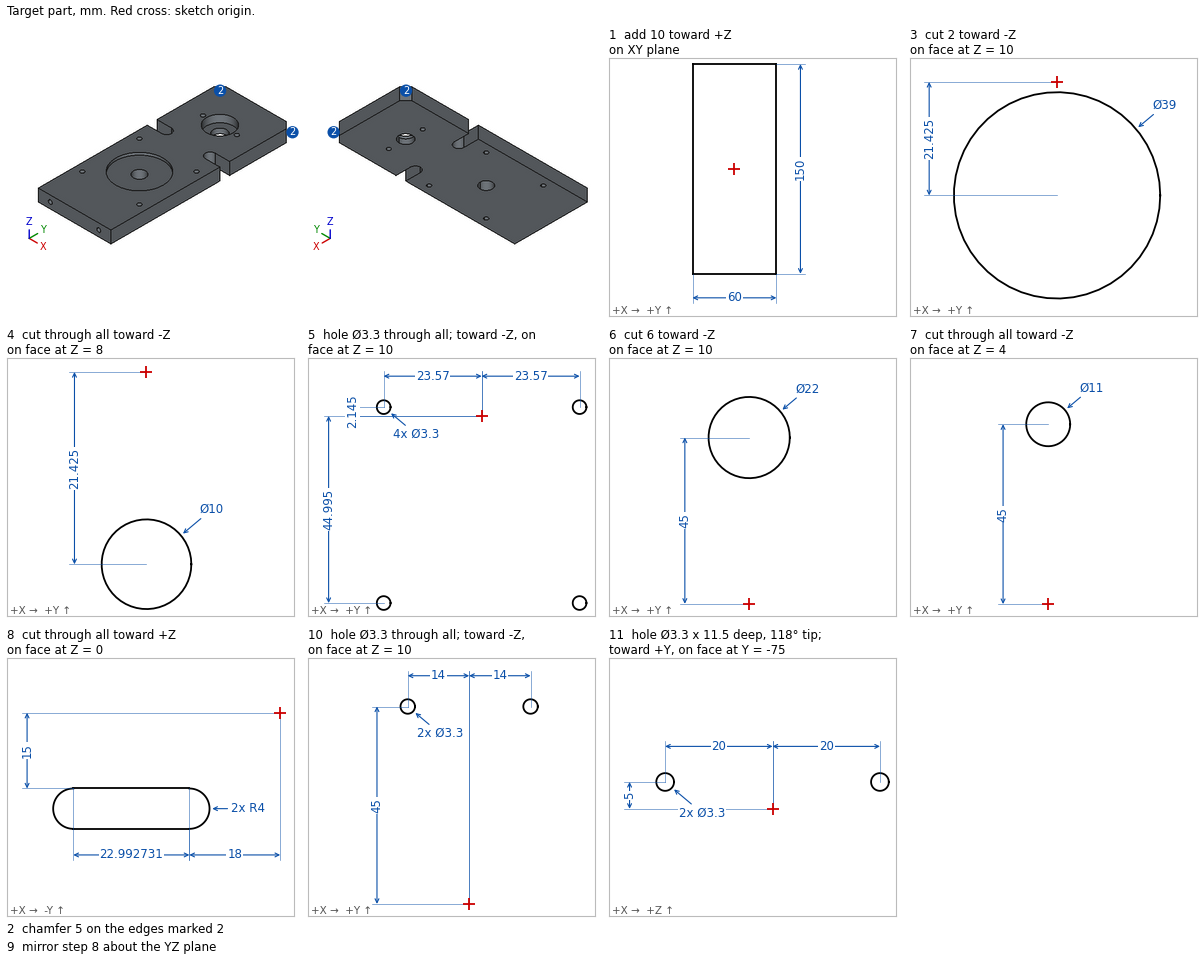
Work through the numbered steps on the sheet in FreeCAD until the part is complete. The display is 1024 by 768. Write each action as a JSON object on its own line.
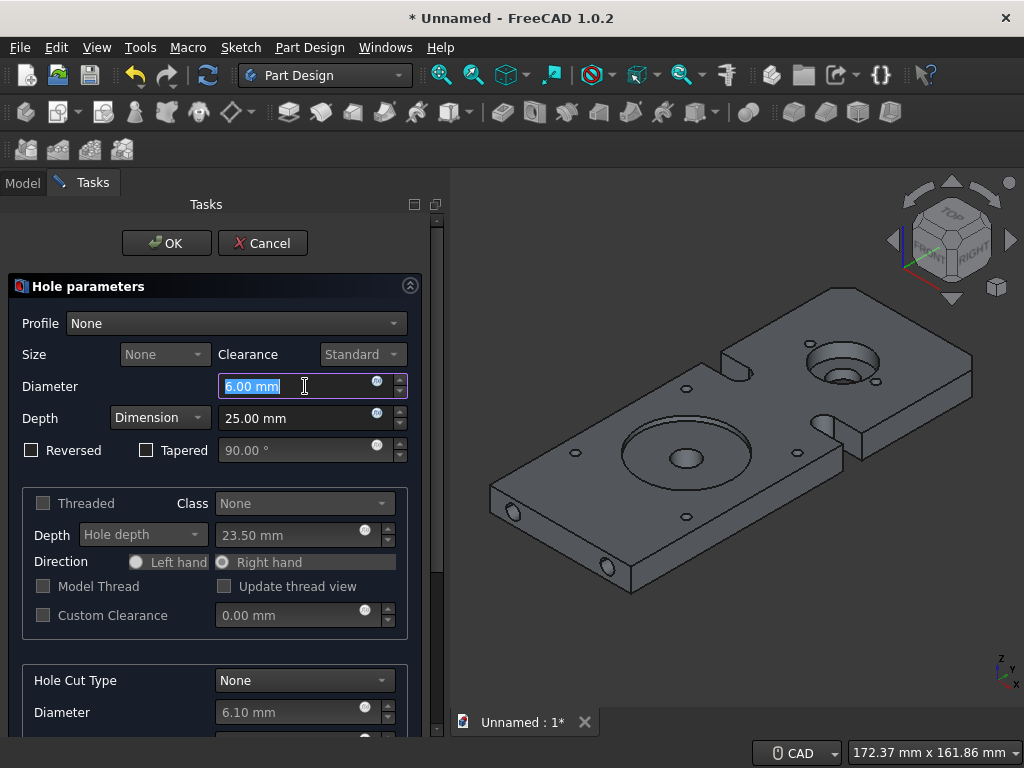
{"action": "type", "text": "3.3"}
{"action": "key", "text": "Tab"}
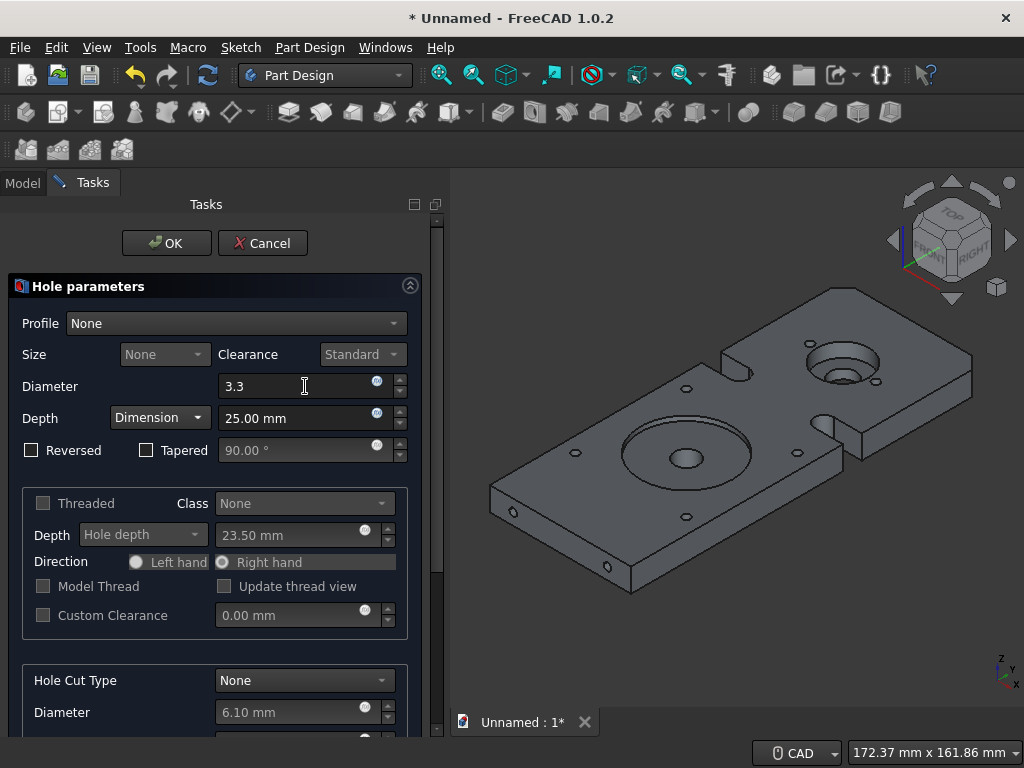
{"action": "triple_click", "coordinate": [305, 418]}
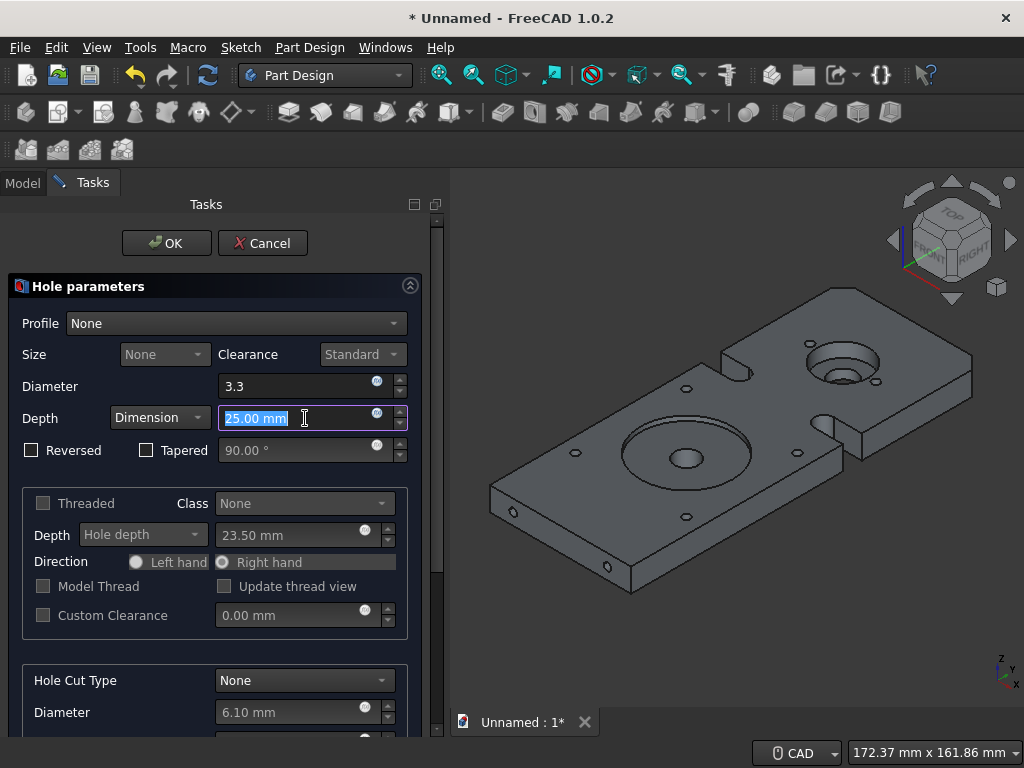
{"action": "type", "text": "11.5"}
{"action": "key", "text": "Tab"}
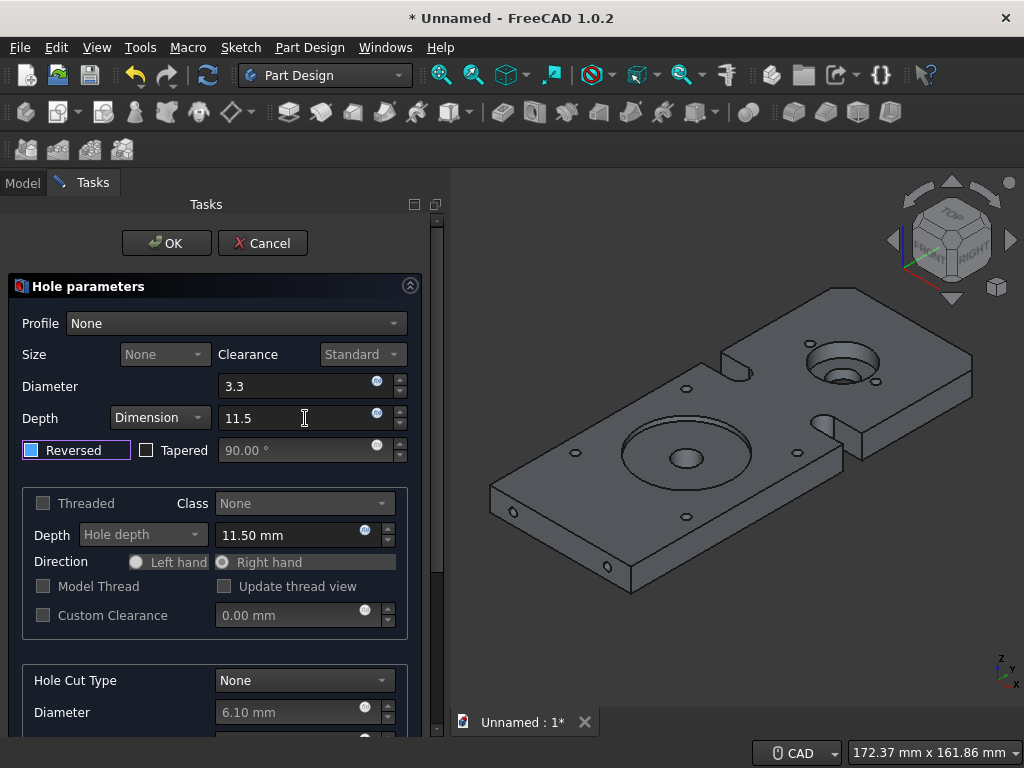
{"action": "left_click", "coordinate": [167, 243]}